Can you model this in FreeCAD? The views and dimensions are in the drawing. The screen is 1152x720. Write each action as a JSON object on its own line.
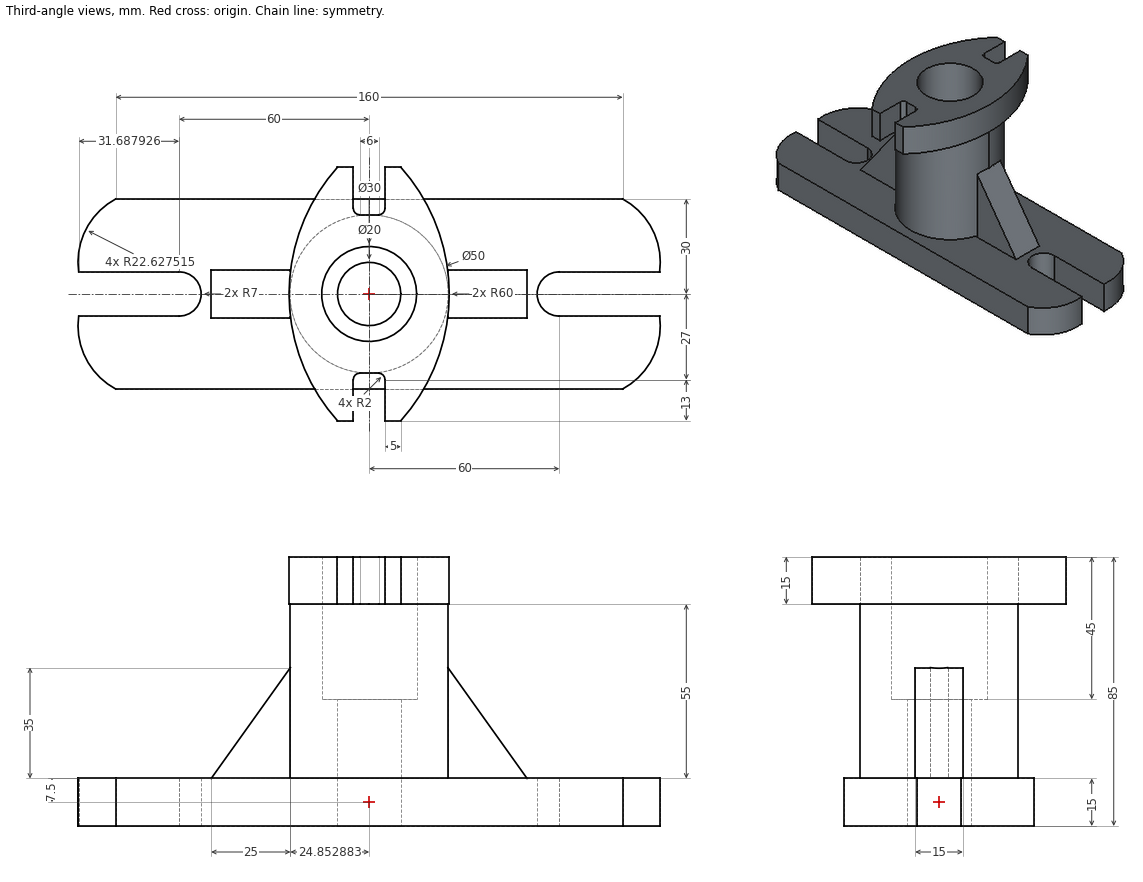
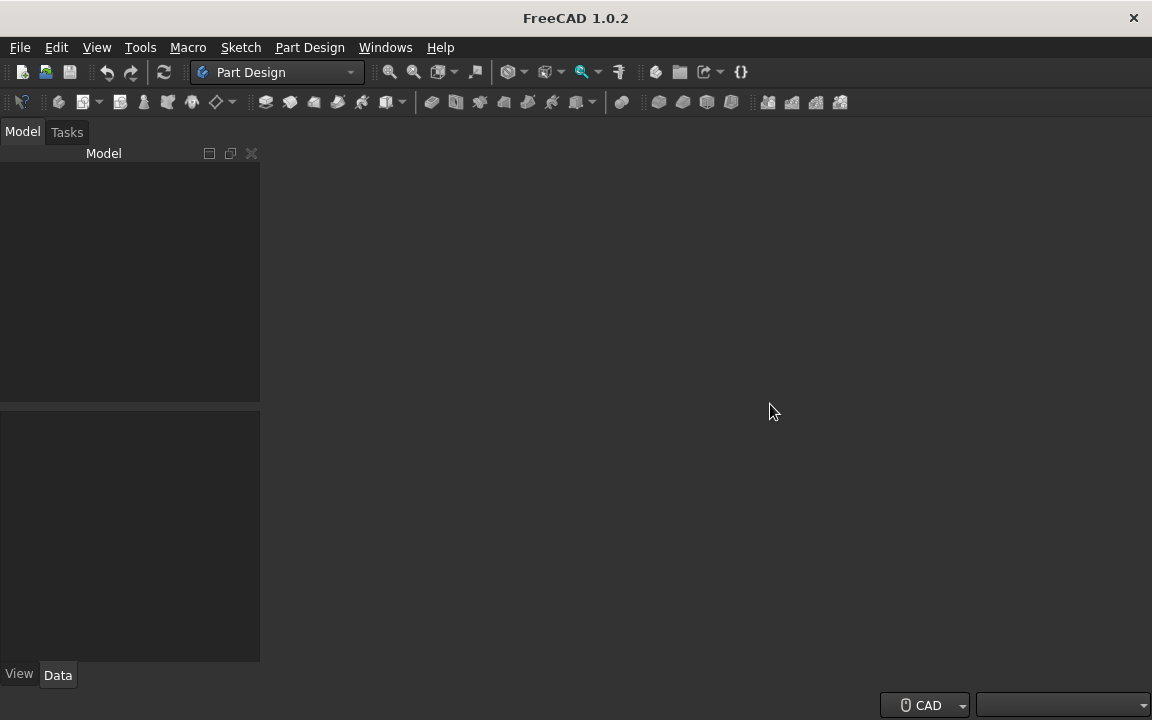
{"action": "key", "text": "ctrl+n"}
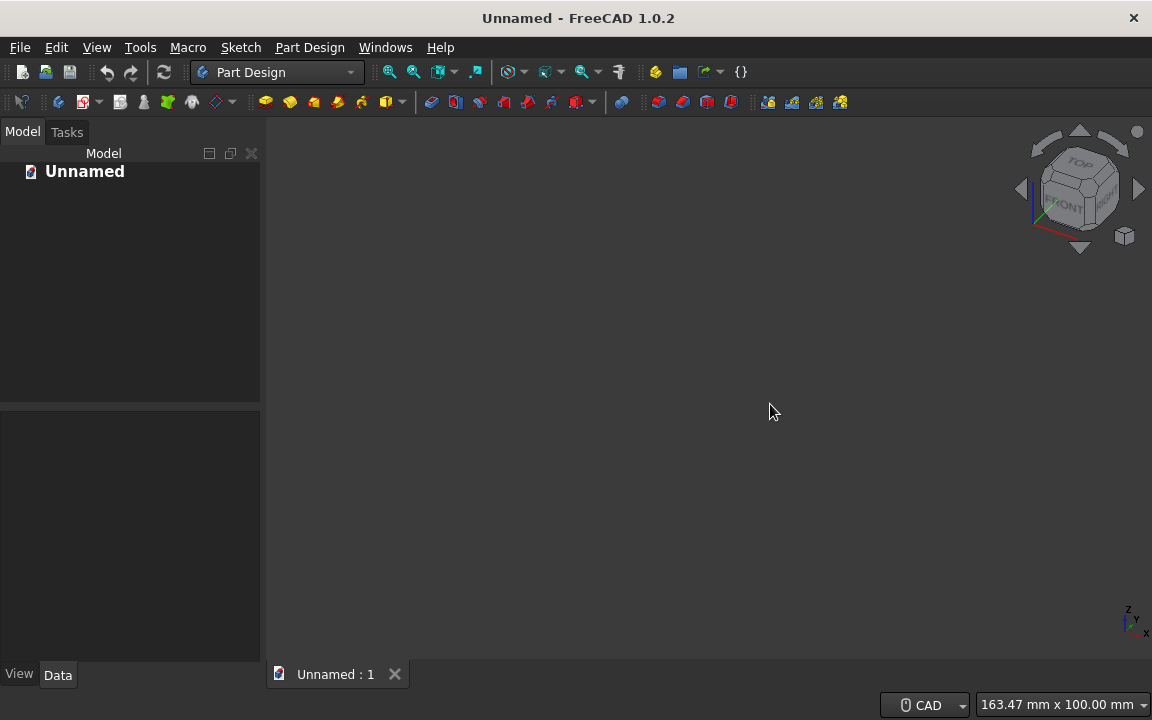
{"action": "left_click", "coordinate": [84, 102]}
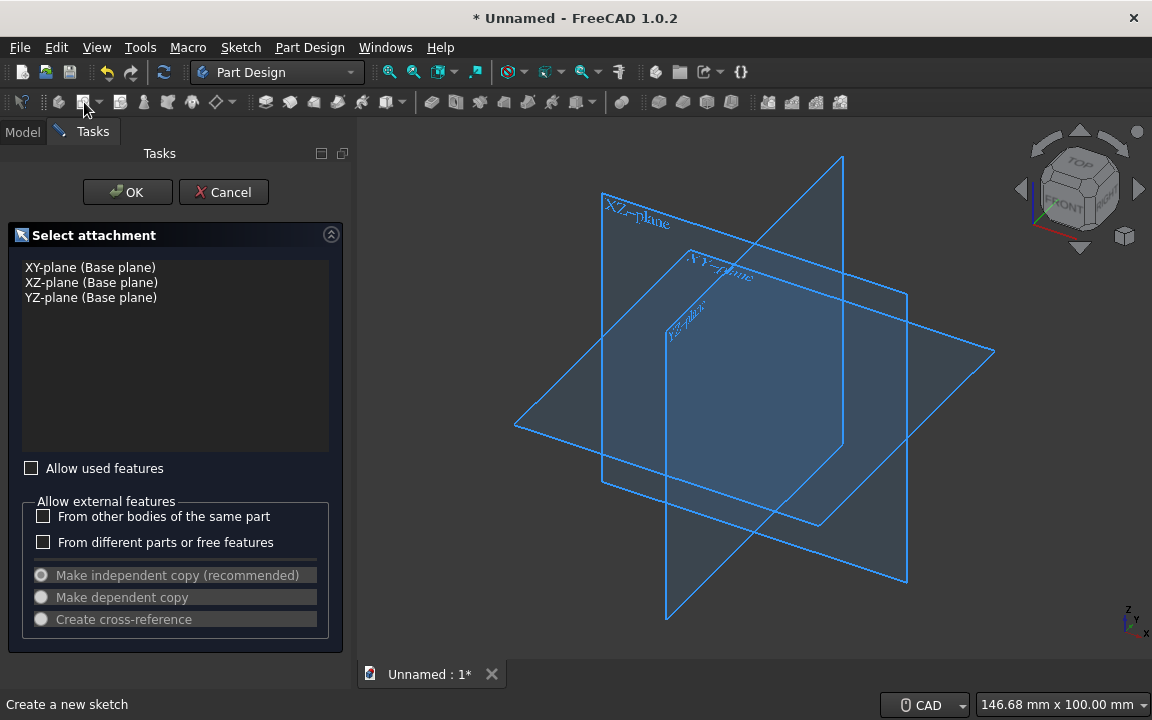
{"action": "left_click", "coordinate": [82, 268]}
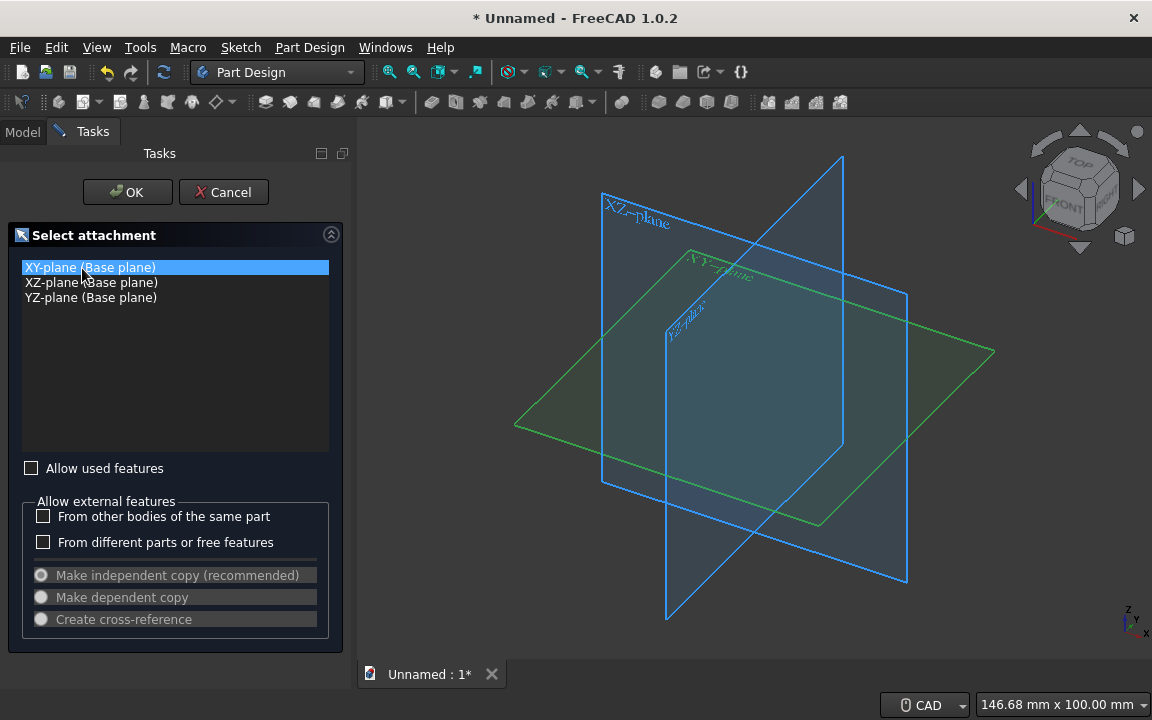
{"action": "left_click", "coordinate": [128, 192]}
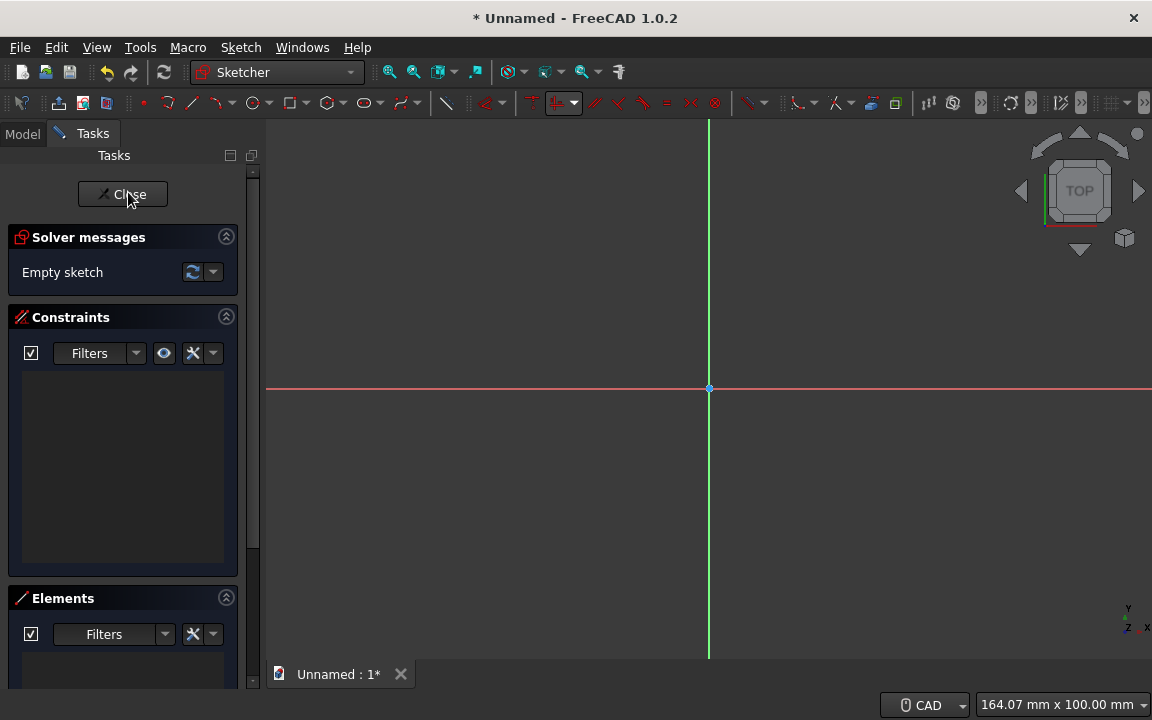
{"action": "scroll", "coordinate": [585, 389], "scroll_direction": "down", "scroll_amount": 4}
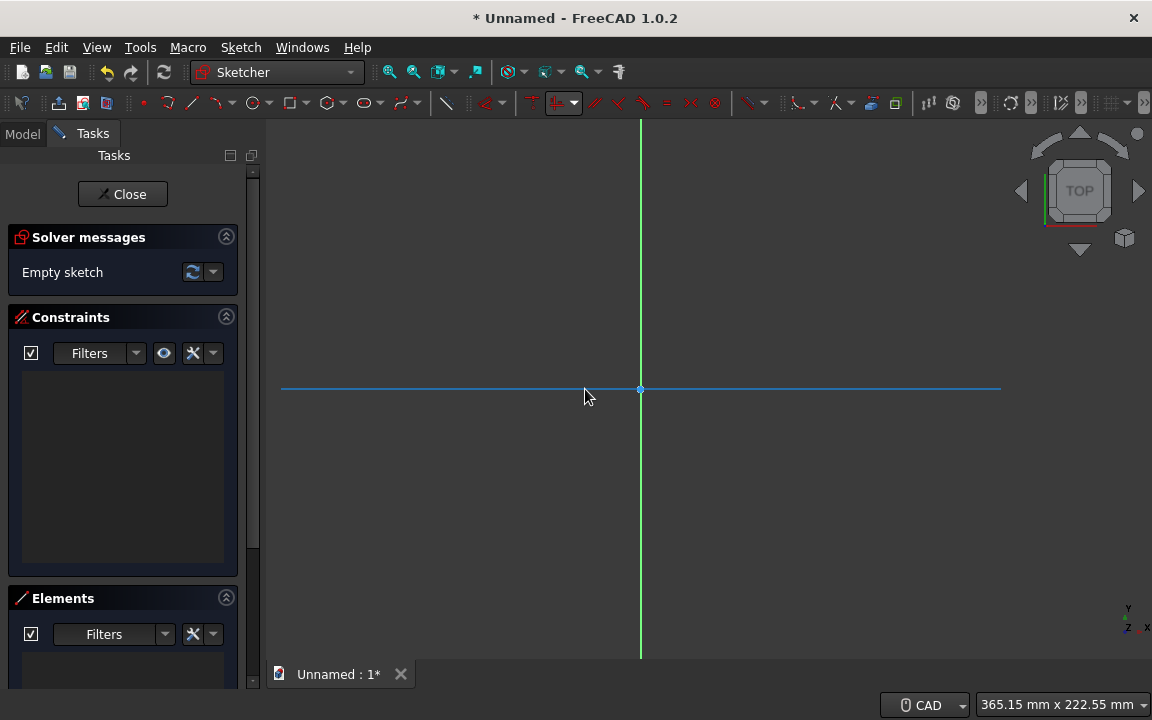
{"action": "key", "text": "g l"}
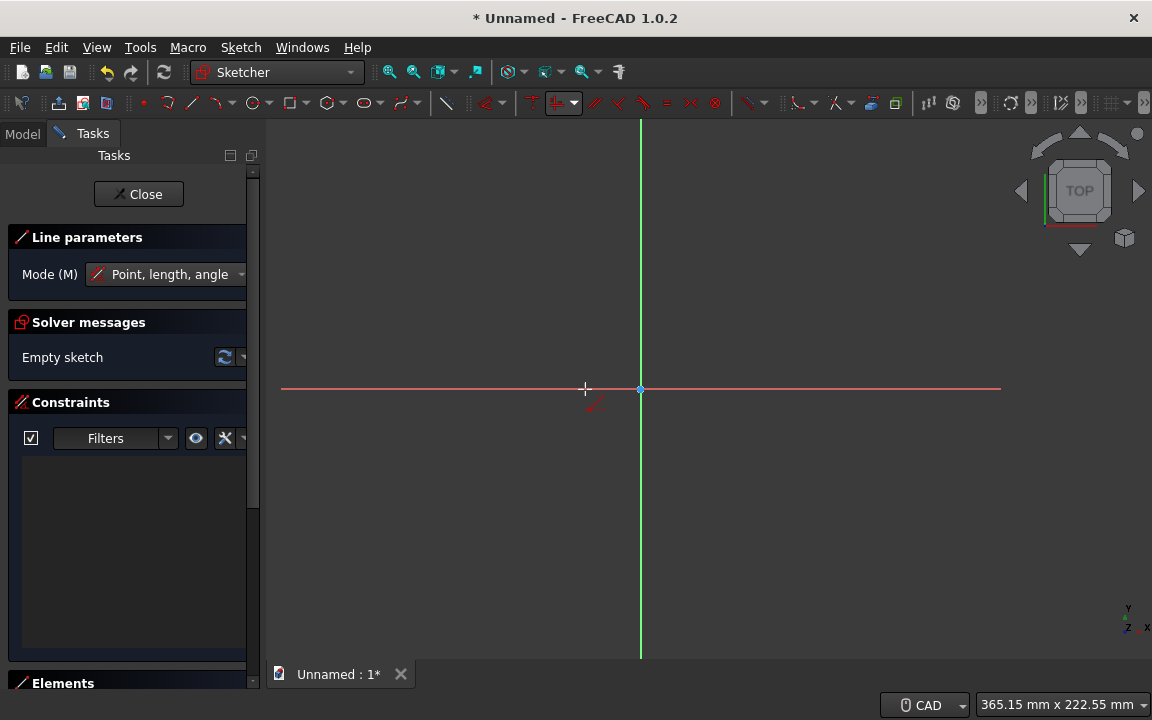
{"action": "left_click", "coordinate": [835, 316]}
{"action": "left_click", "coordinate": [447, 316]}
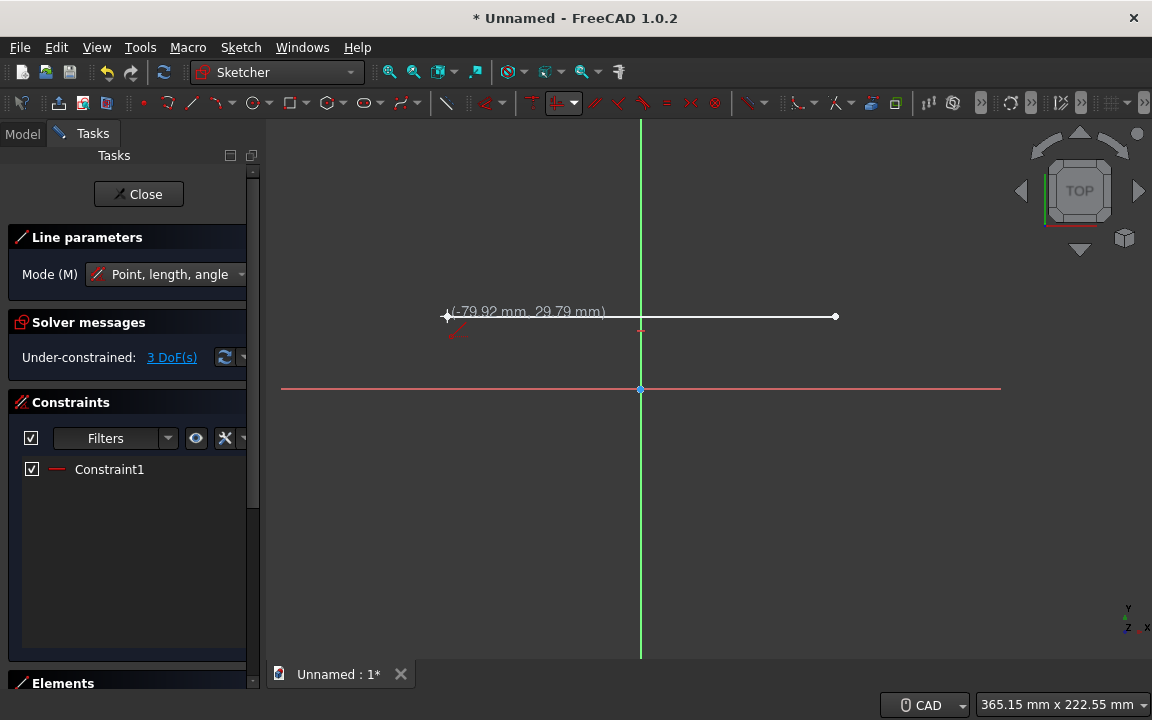
{"action": "left_click", "coordinate": [418, 372]}
{"action": "left_click", "coordinate": [495, 372]}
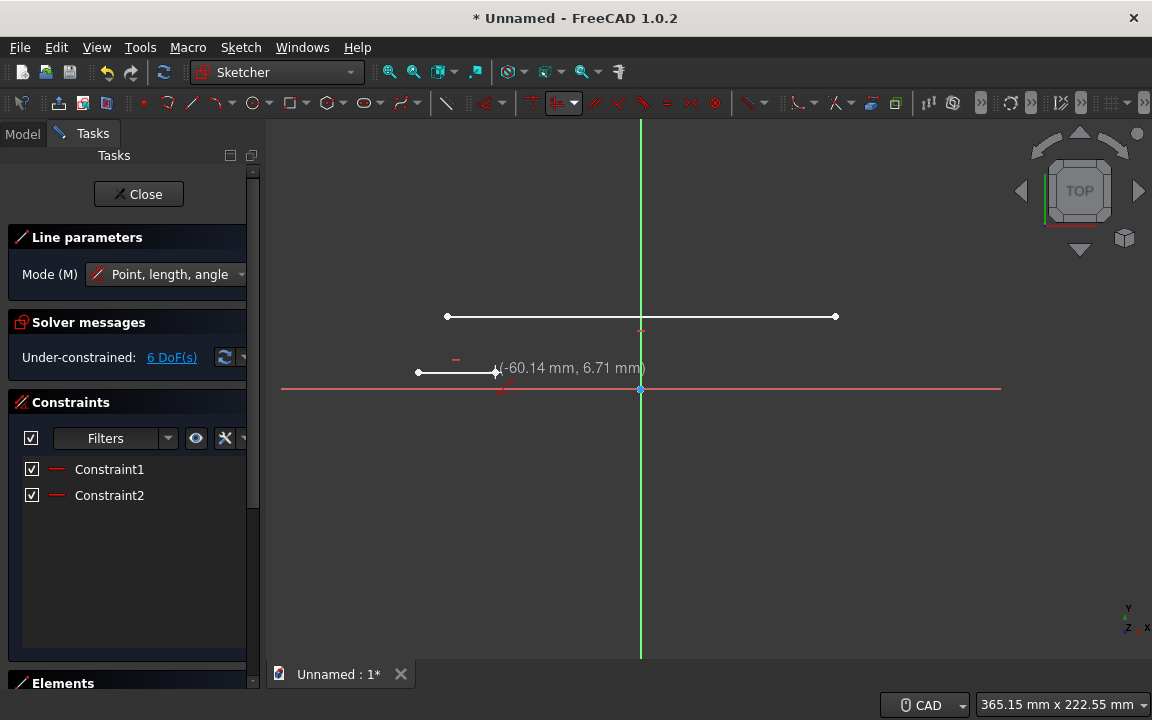
{"action": "left_click", "coordinate": [495, 406]}
{"action": "left_click", "coordinate": [418, 406]}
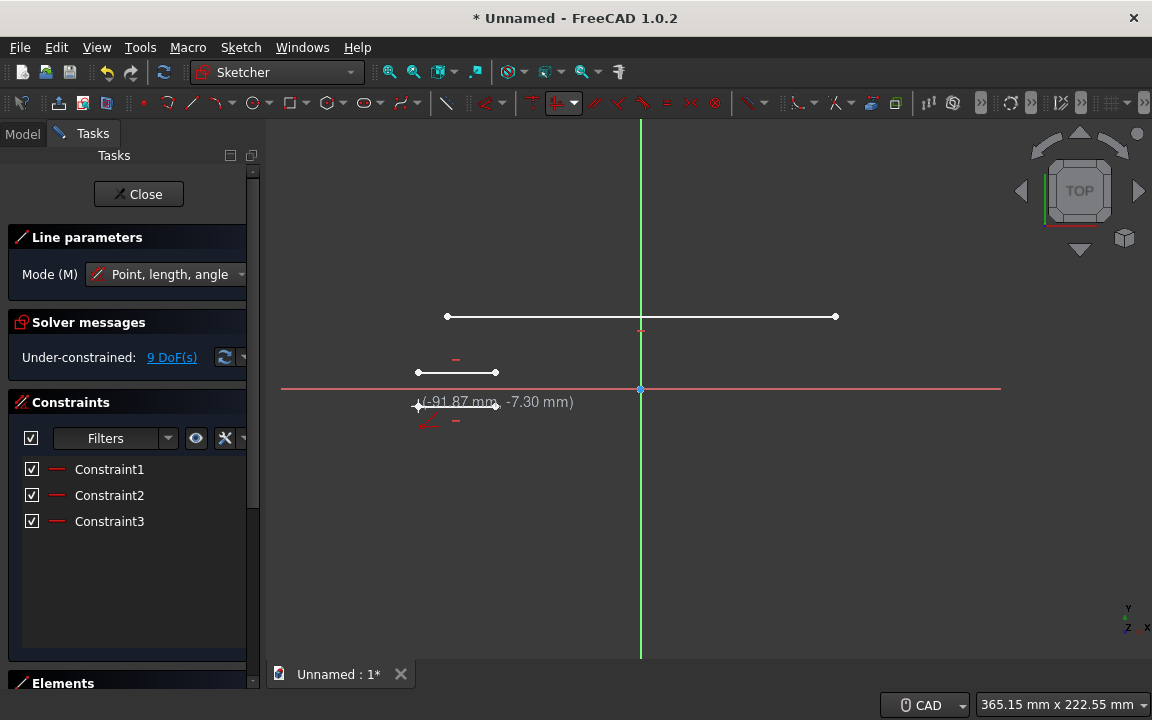
{"action": "left_click", "coordinate": [447, 462]}
{"action": "left_click", "coordinate": [835, 462]}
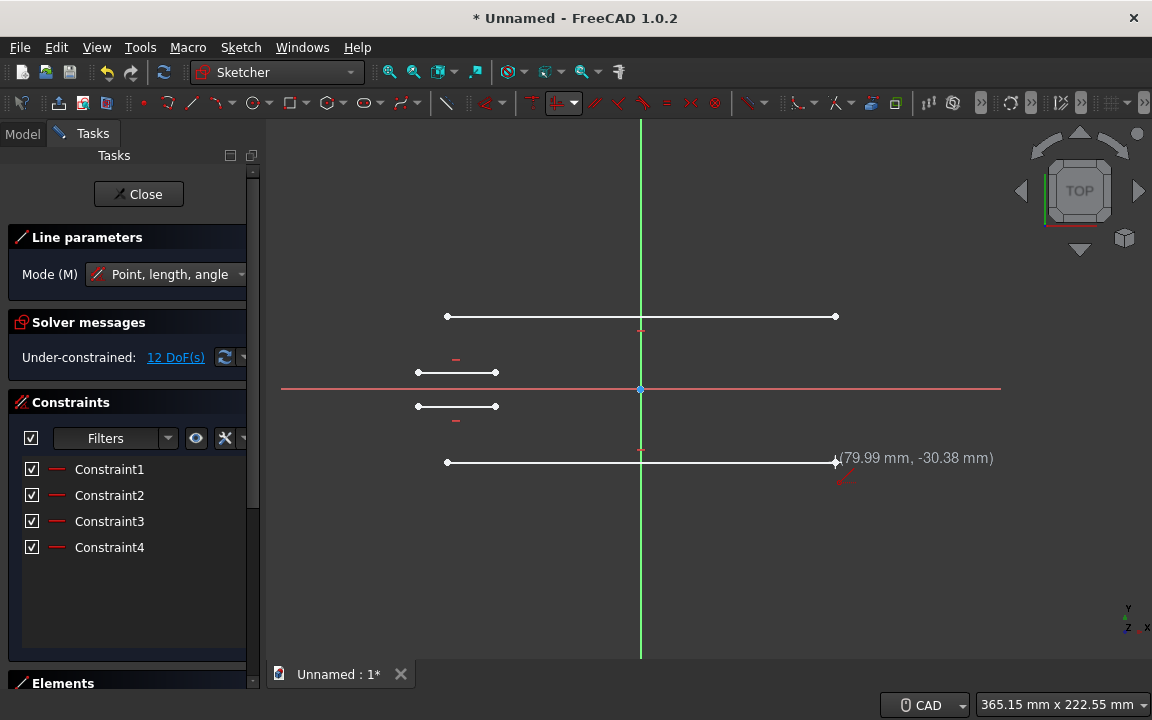
{"action": "left_click", "coordinate": [863, 406]}
{"action": "left_click", "coordinate": [786, 406]}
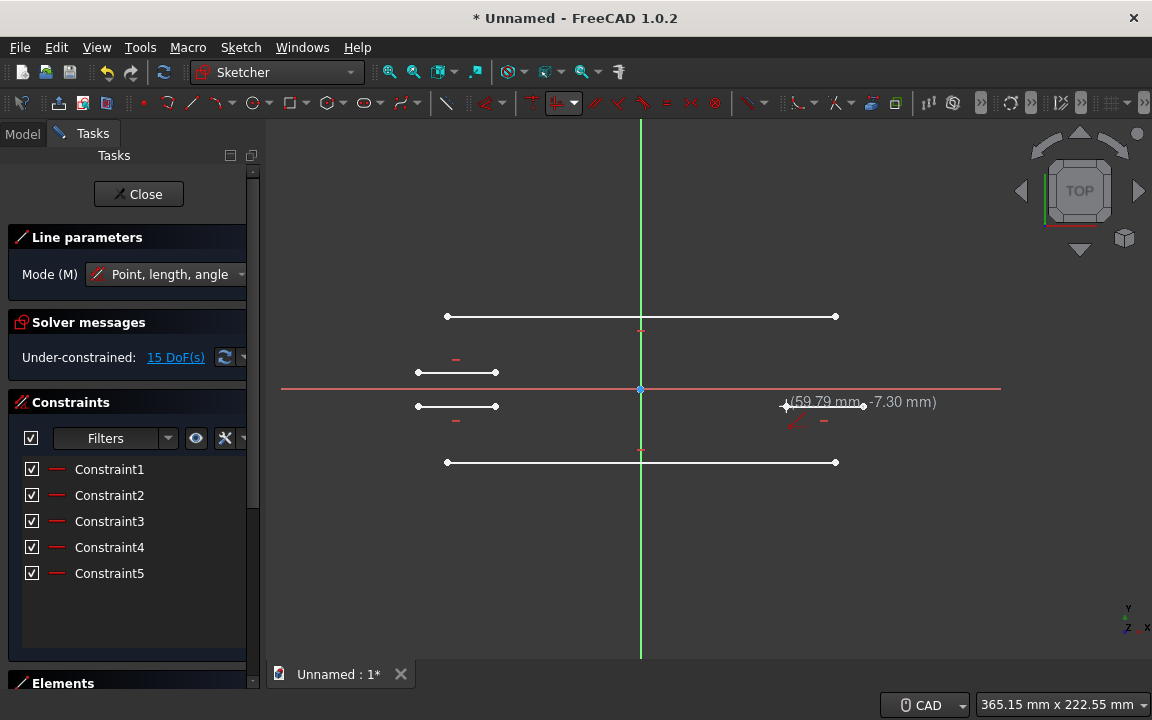
{"action": "left_click", "coordinate": [786, 372]}
{"action": "left_click", "coordinate": [863, 372]}